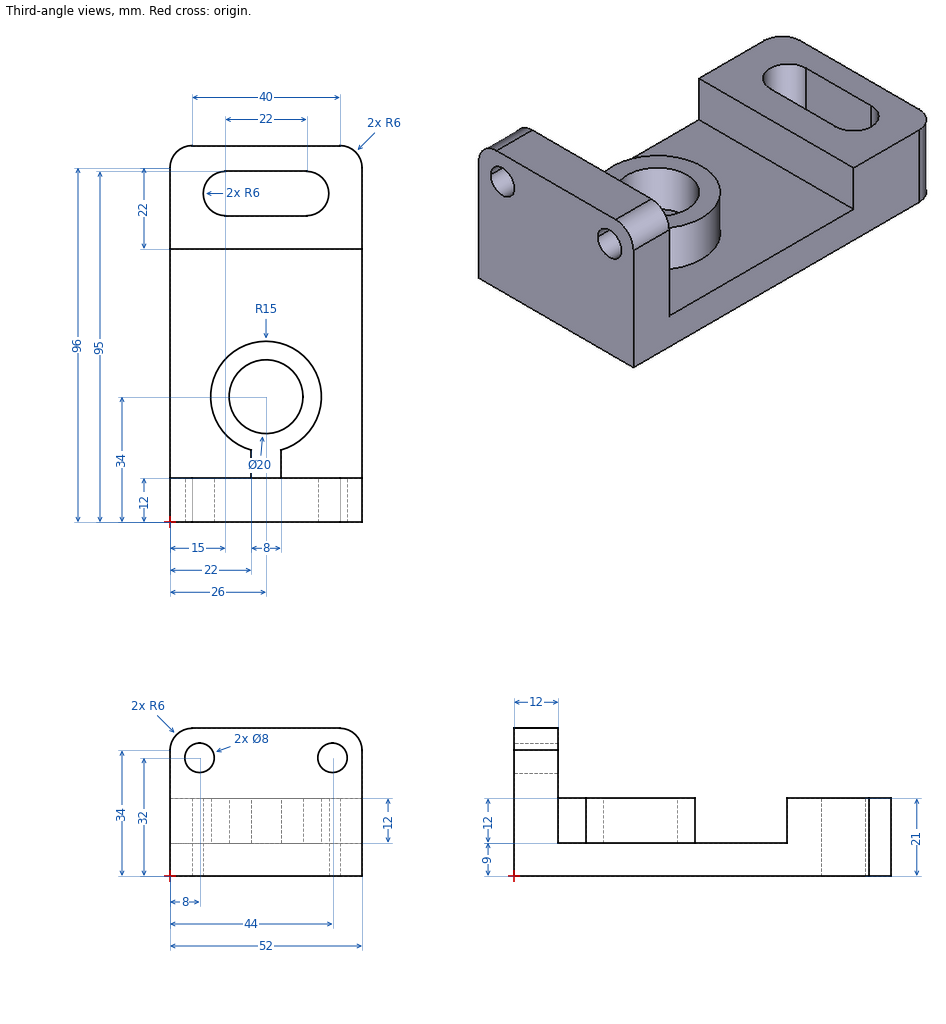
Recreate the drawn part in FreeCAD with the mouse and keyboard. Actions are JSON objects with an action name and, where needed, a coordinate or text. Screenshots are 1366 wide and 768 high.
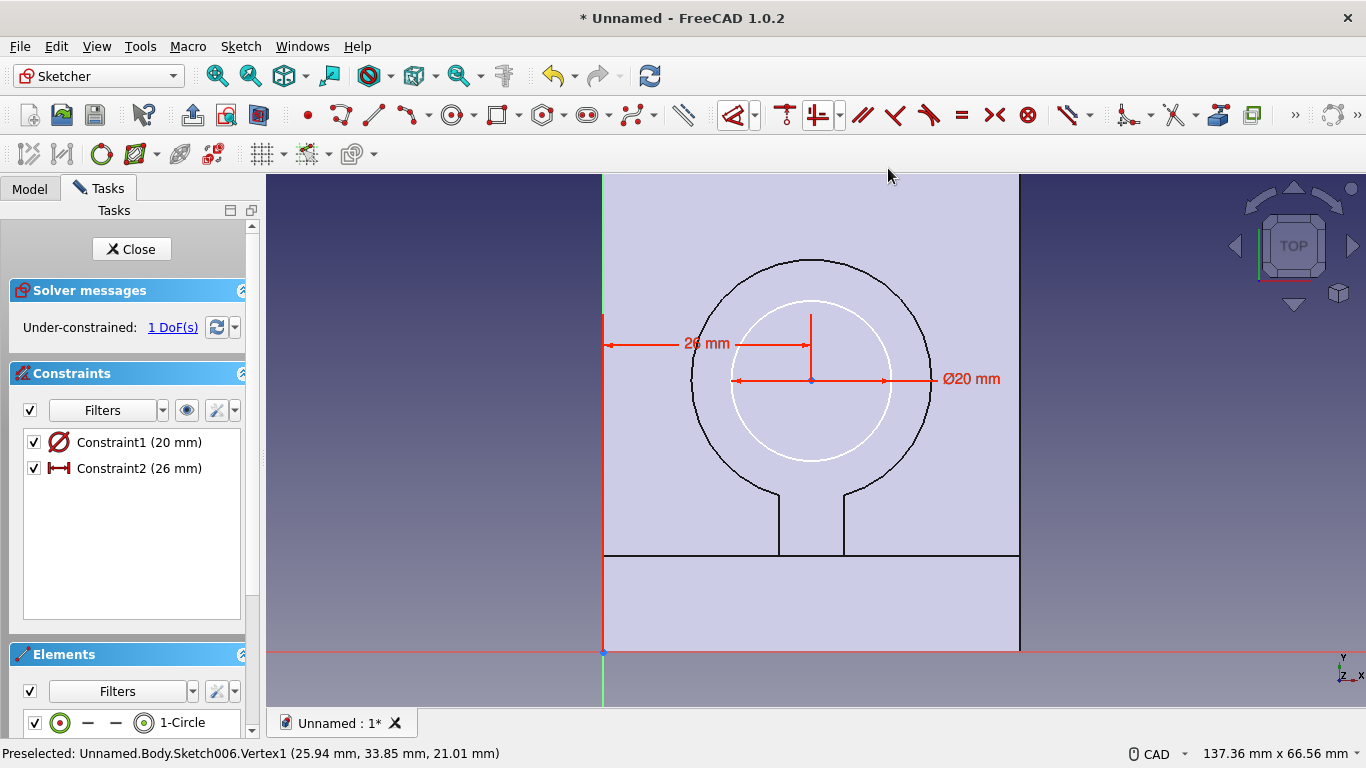
{"action": "left_click", "coordinate": [811, 381]}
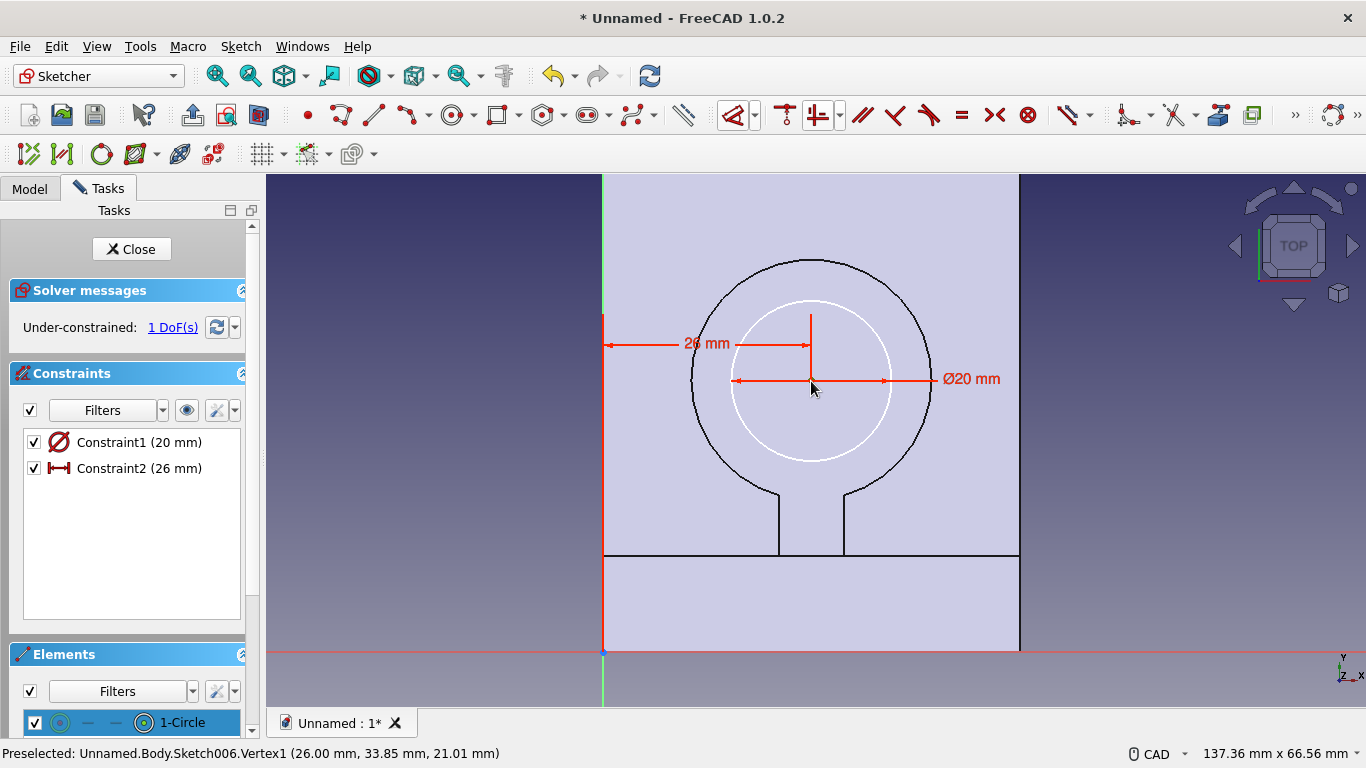
{"action": "key", "text": "i"}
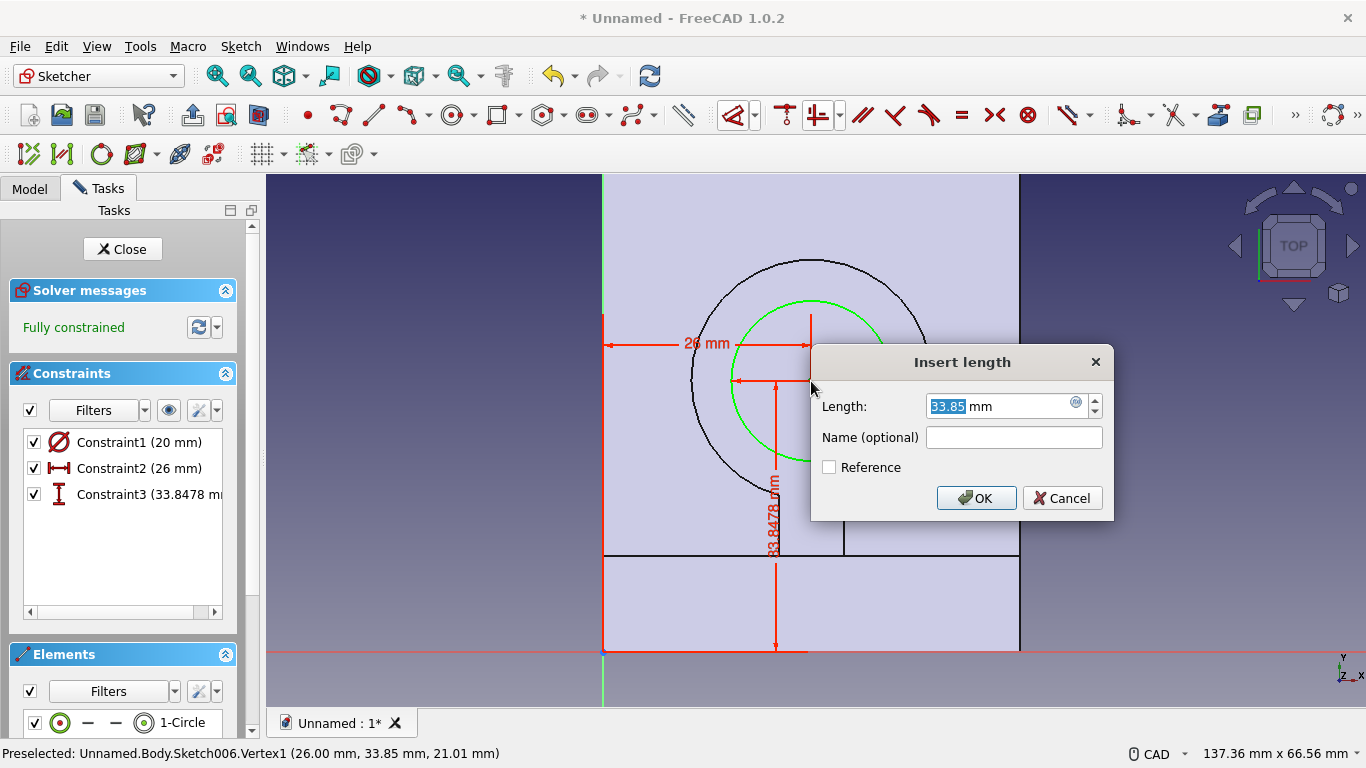
{"action": "type", "text": "34"}
{"action": "key", "text": "Return"}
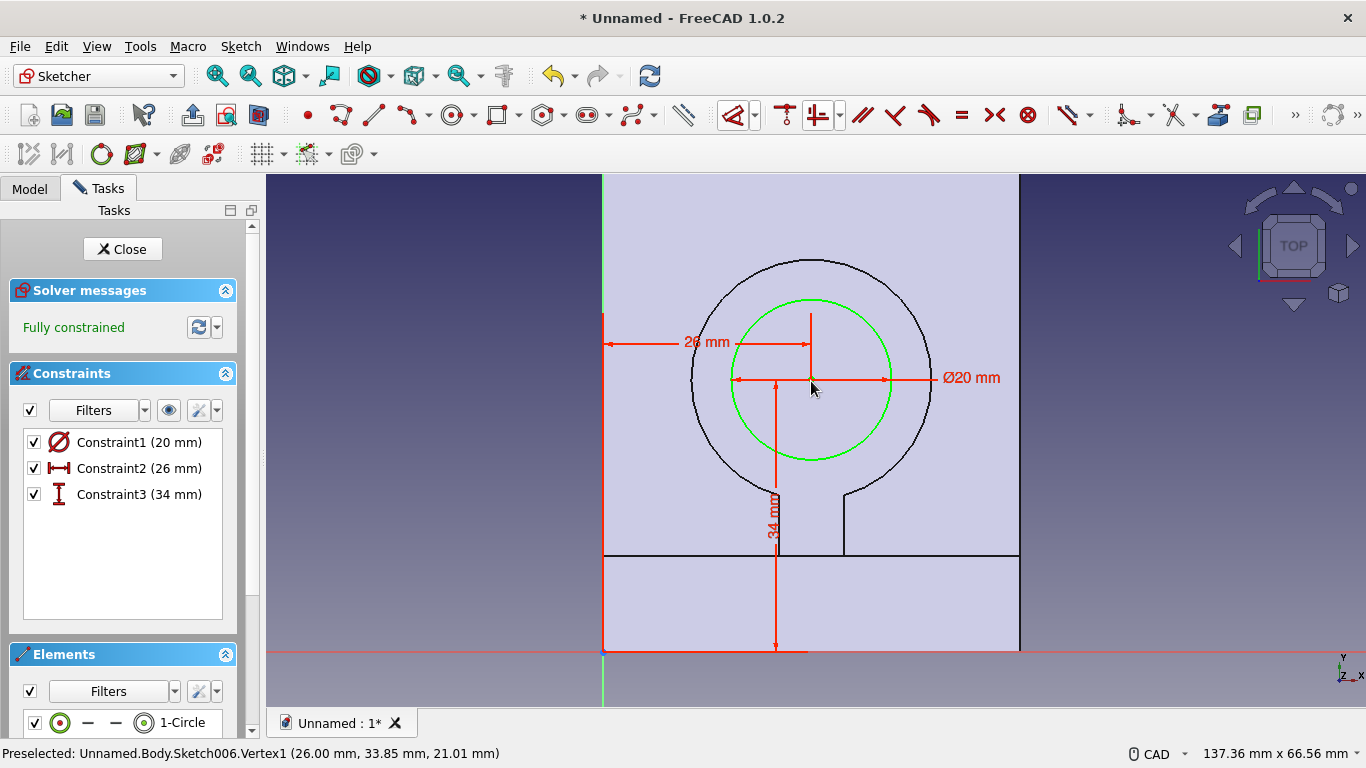
{"action": "left_click", "coordinate": [123, 249]}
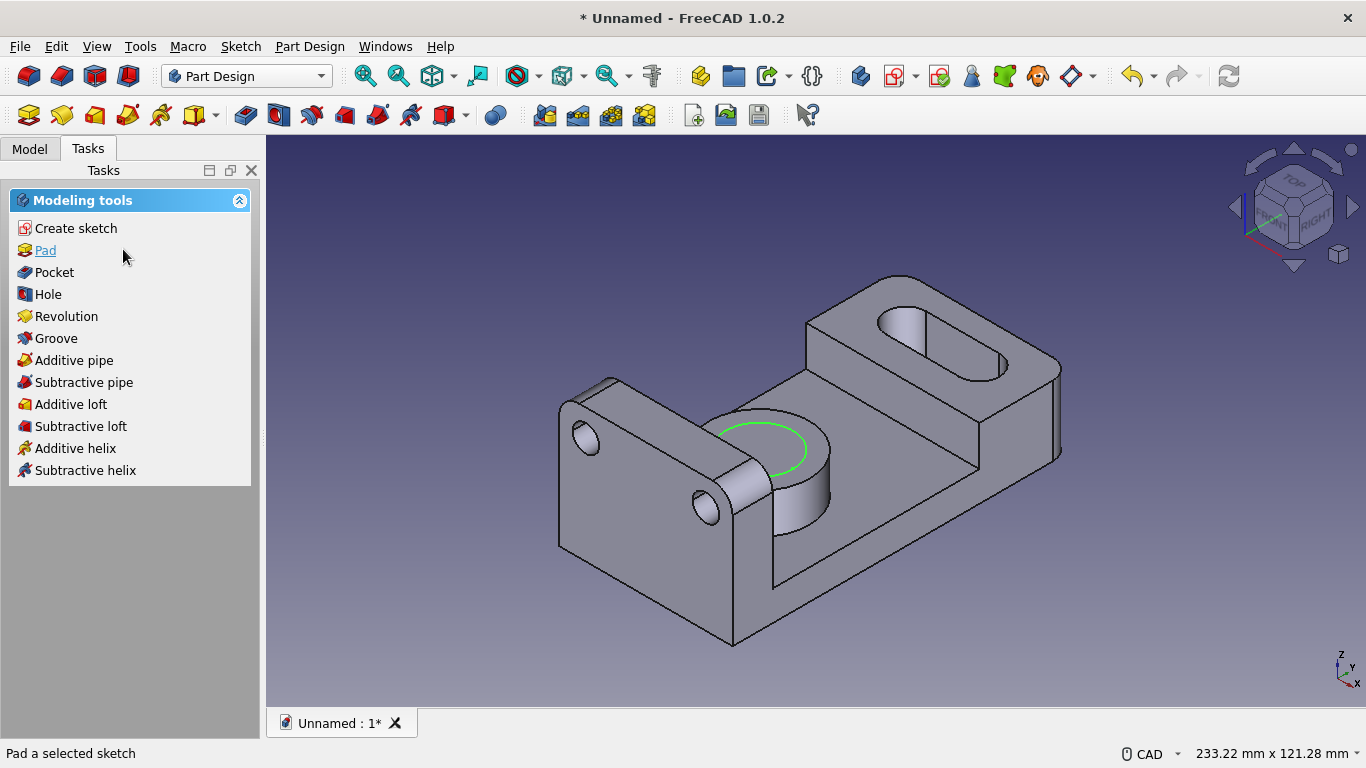
{"action": "left_click", "coordinate": [246, 116]}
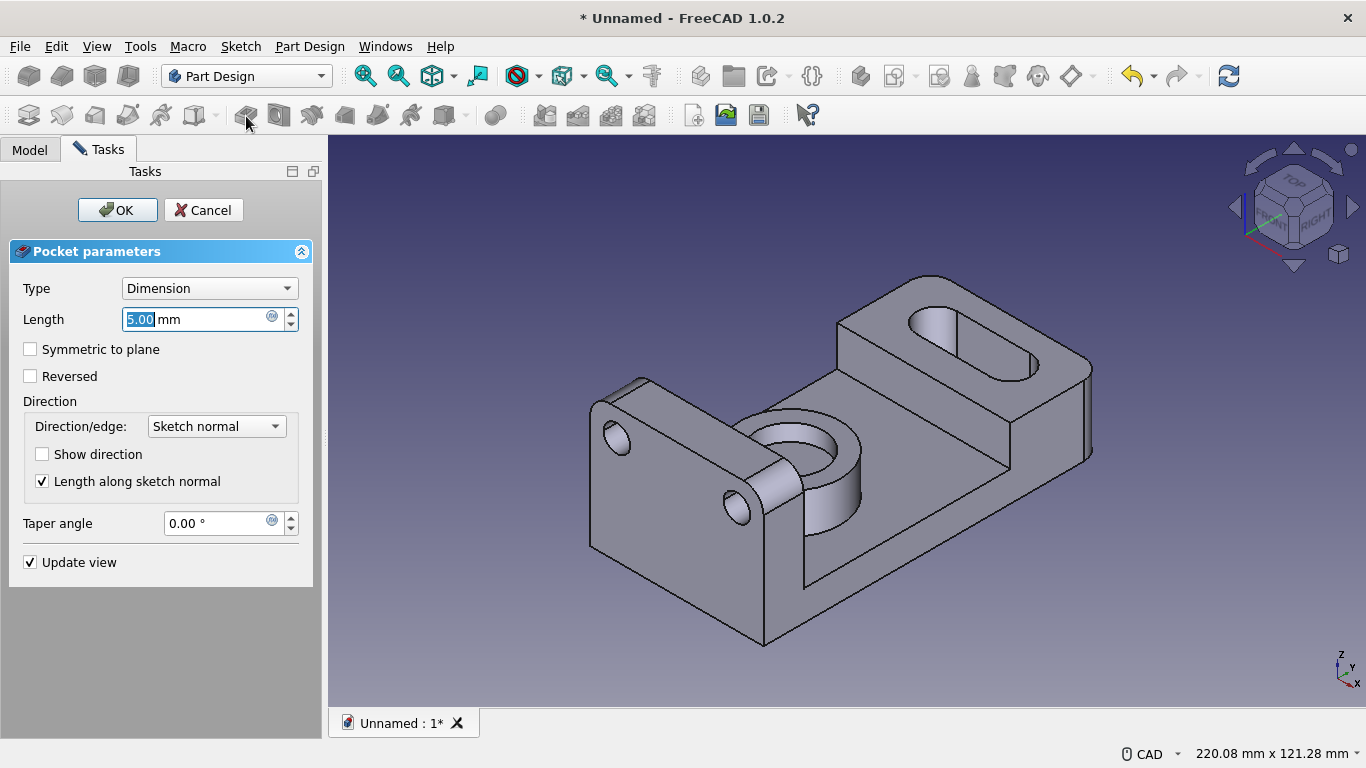
{"action": "type", "text": "12"}
{"action": "key", "text": "Tab"}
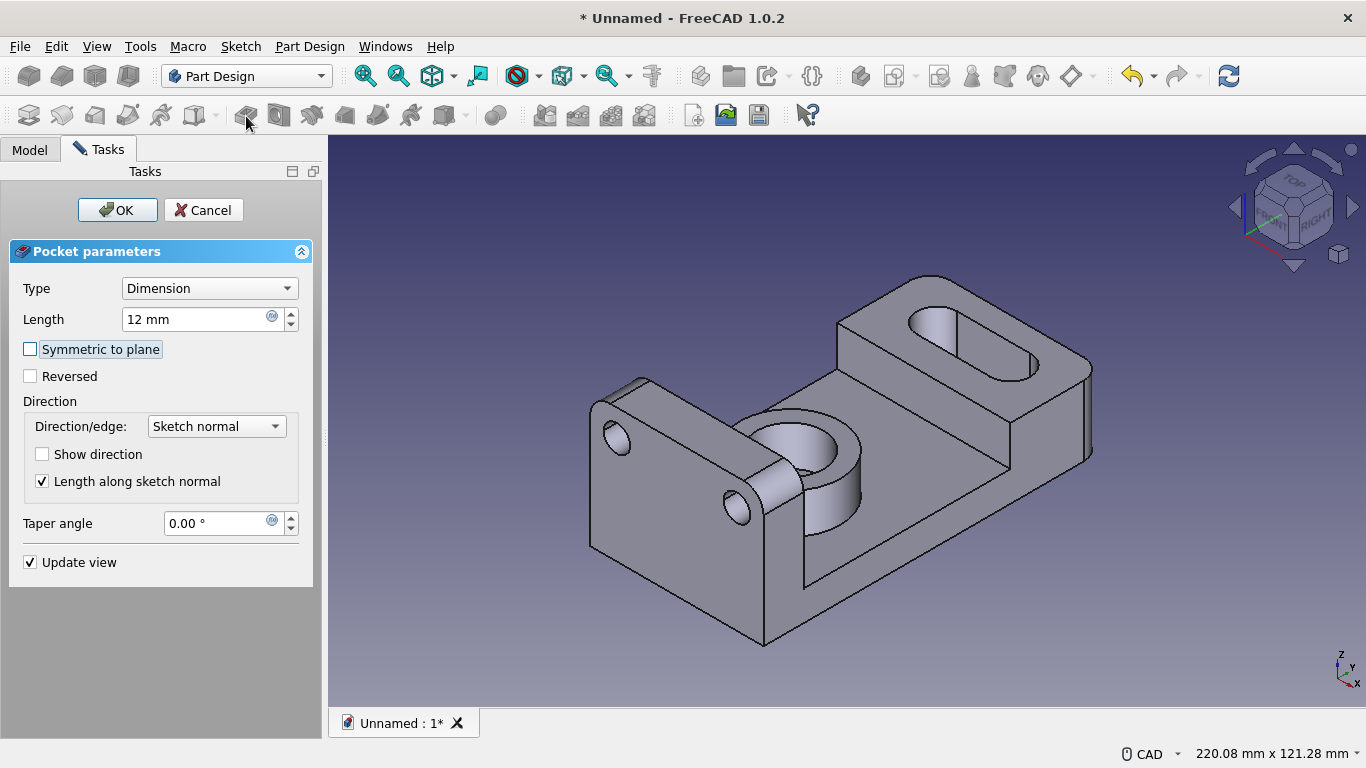
{"action": "left_click", "coordinate": [118, 210]}